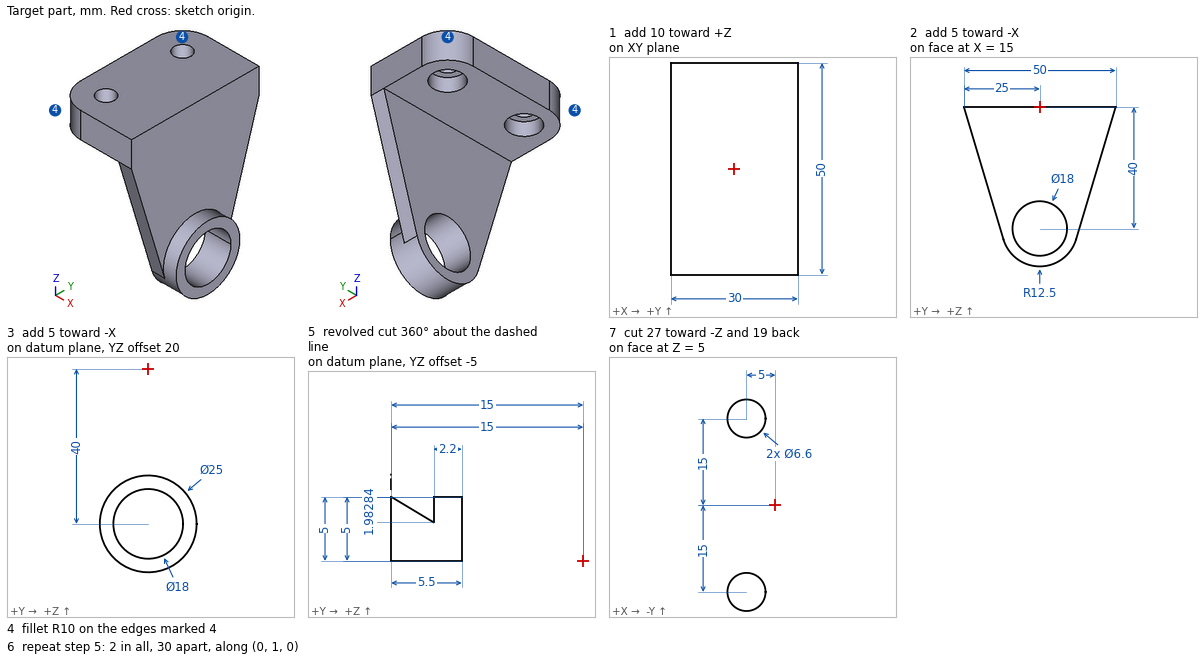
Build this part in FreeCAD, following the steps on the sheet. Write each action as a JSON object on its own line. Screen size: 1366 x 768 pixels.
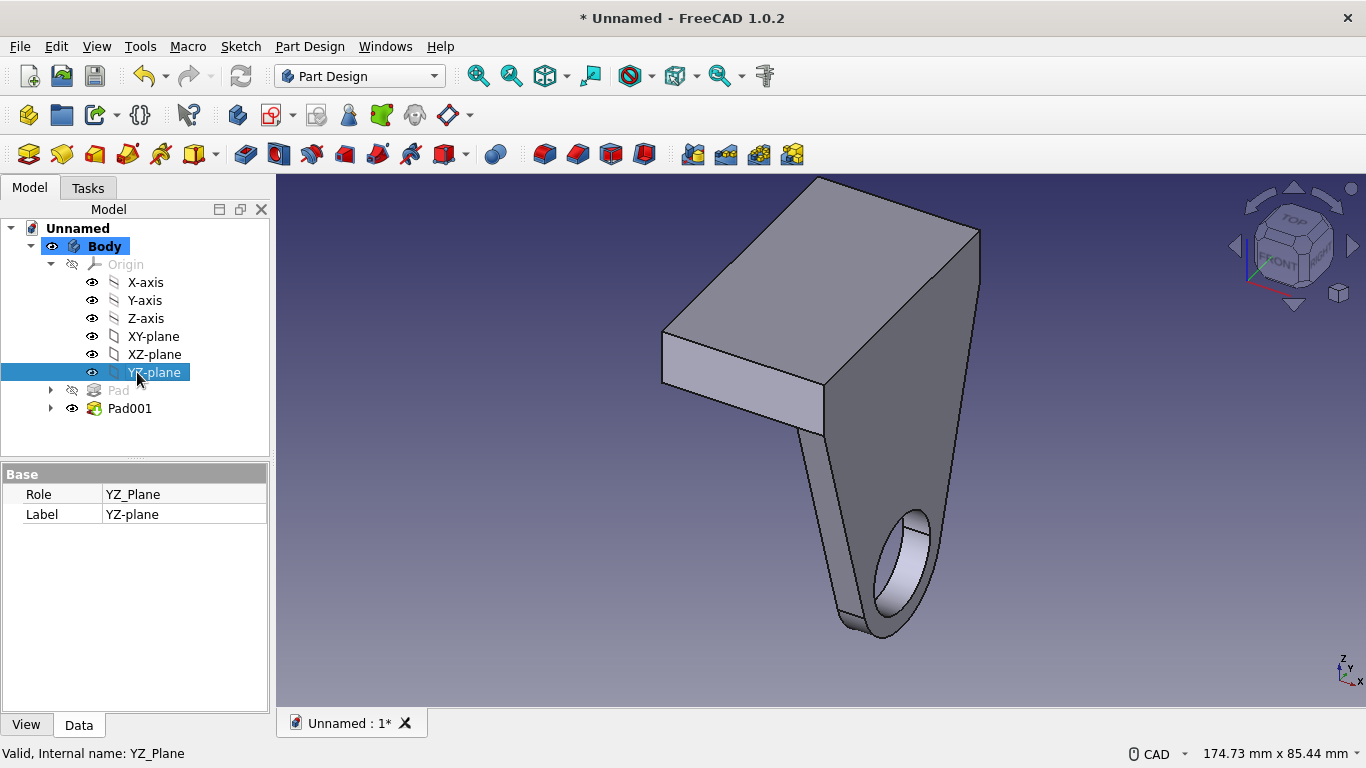
{"action": "left_click", "coordinate": [448, 116]}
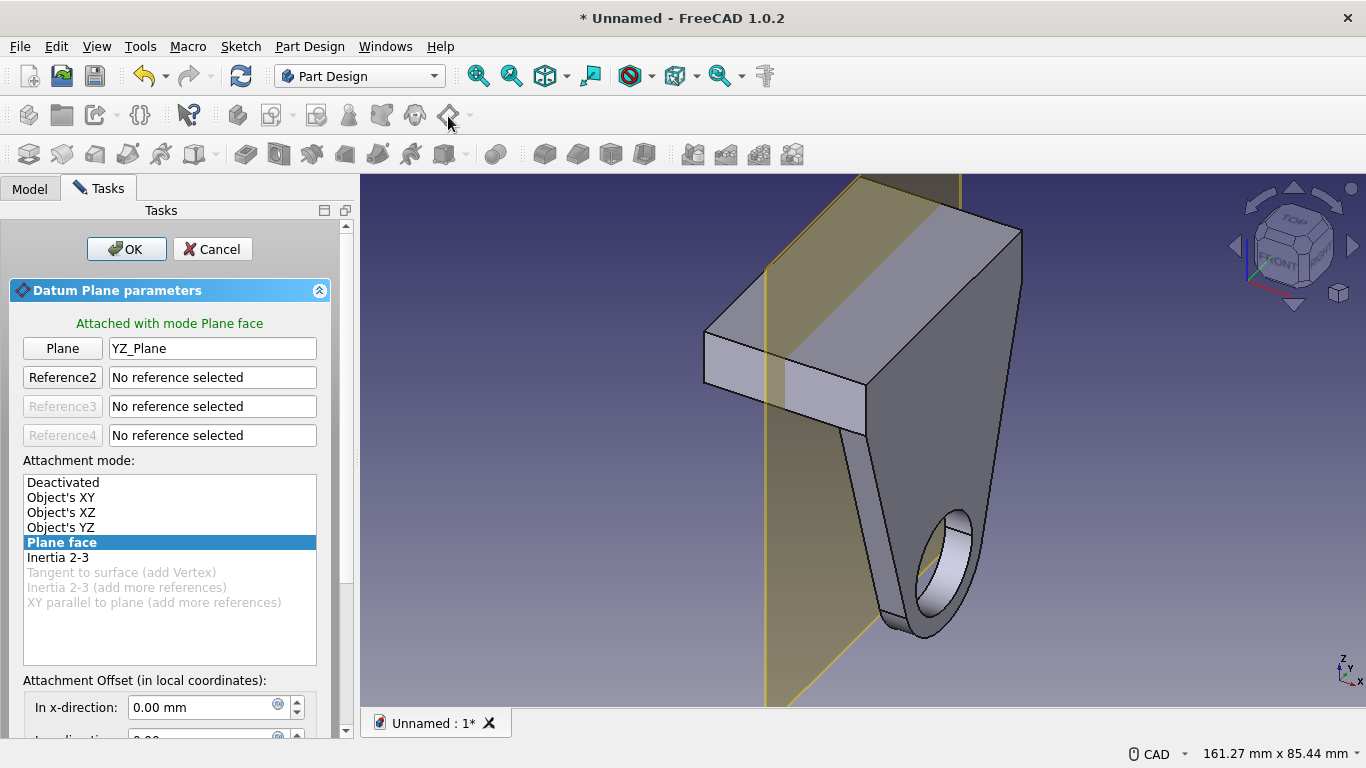
{"action": "scroll", "coordinate": [346, 479], "scroll_direction": "down", "scroll_amount": 2}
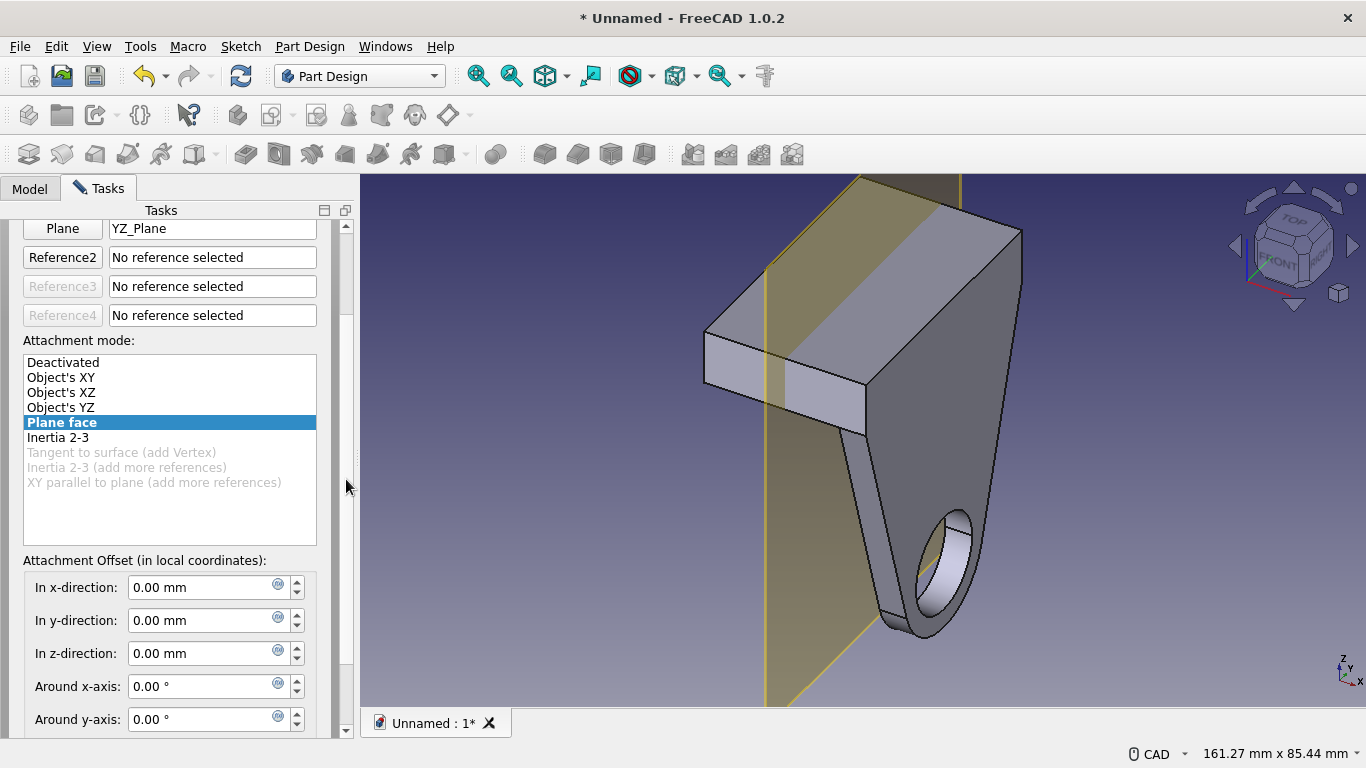
{"action": "triple_click", "coordinate": [210, 654]}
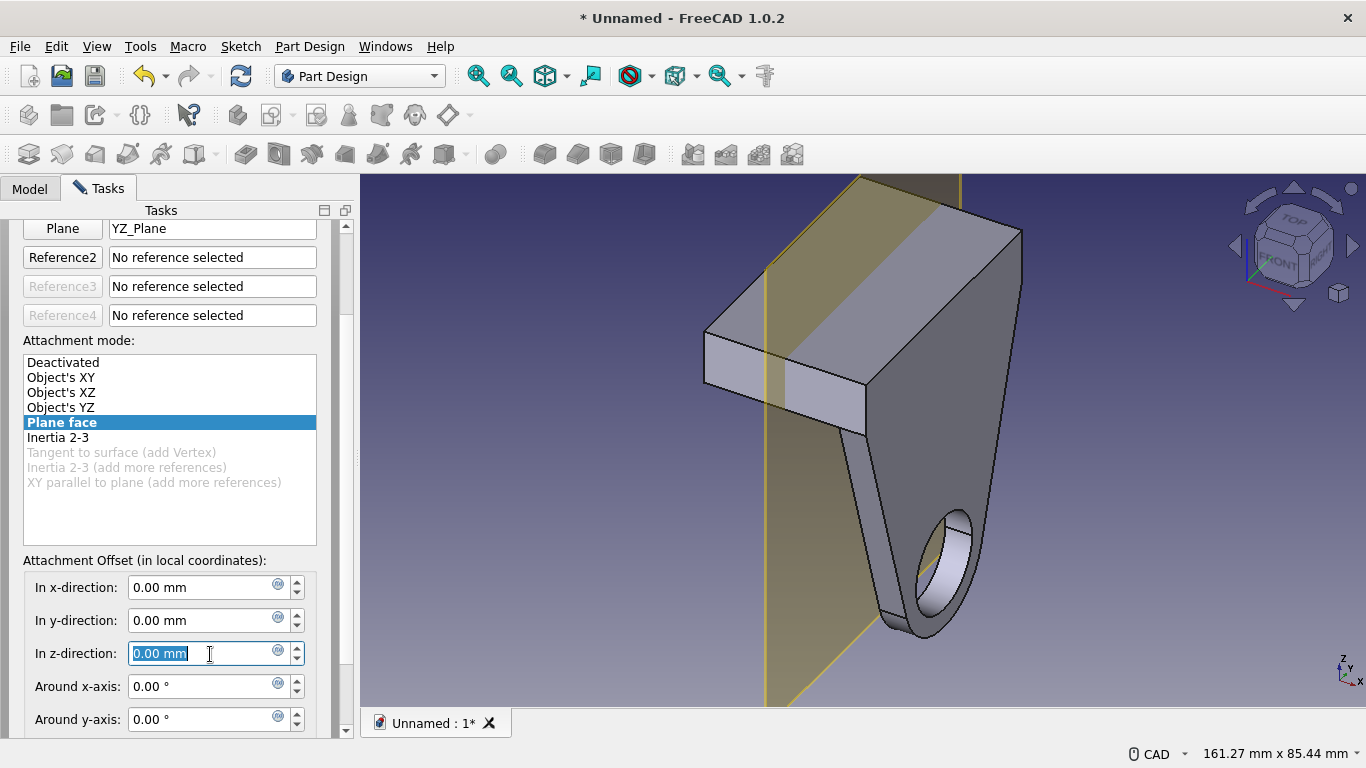
{"action": "type", "text": "20"}
{"action": "key", "text": "Tab"}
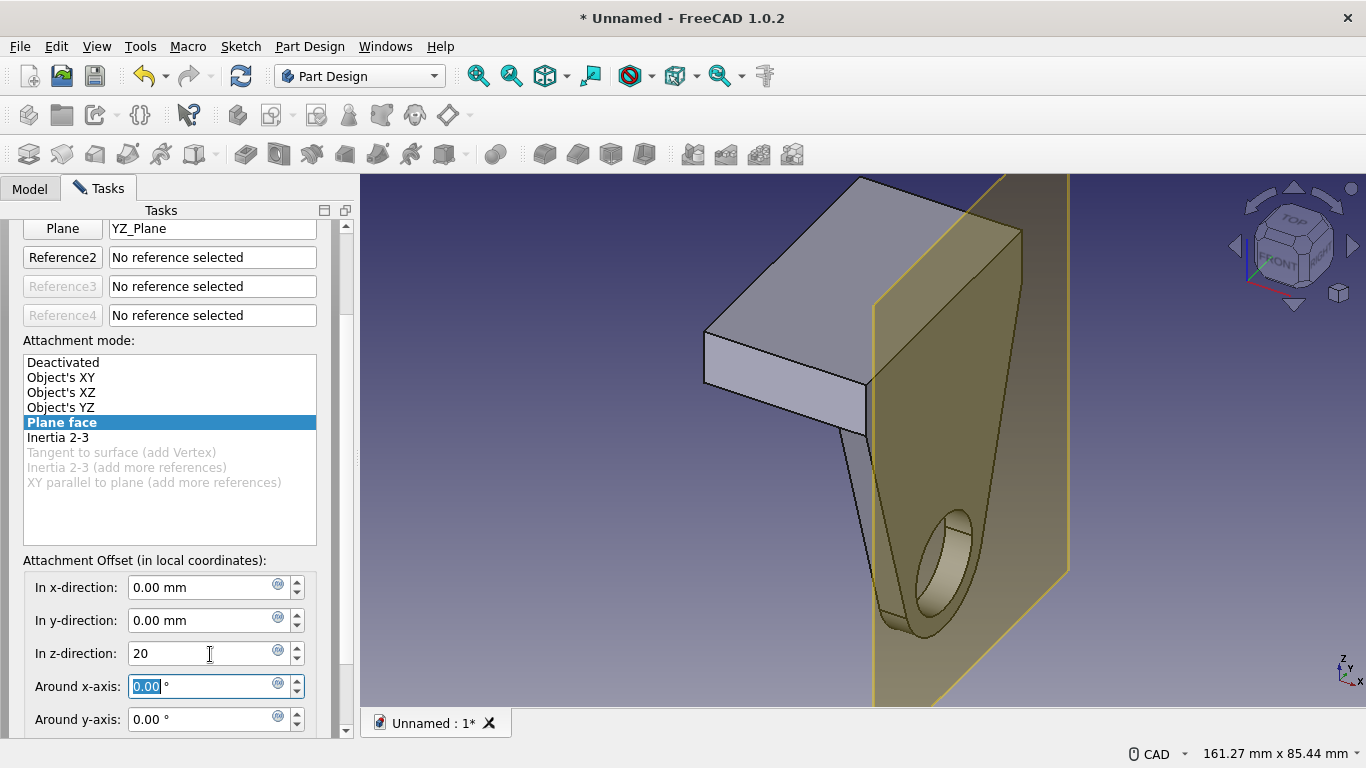
{"action": "scroll", "coordinate": [346, 479], "scroll_direction": "up", "scroll_amount": 3}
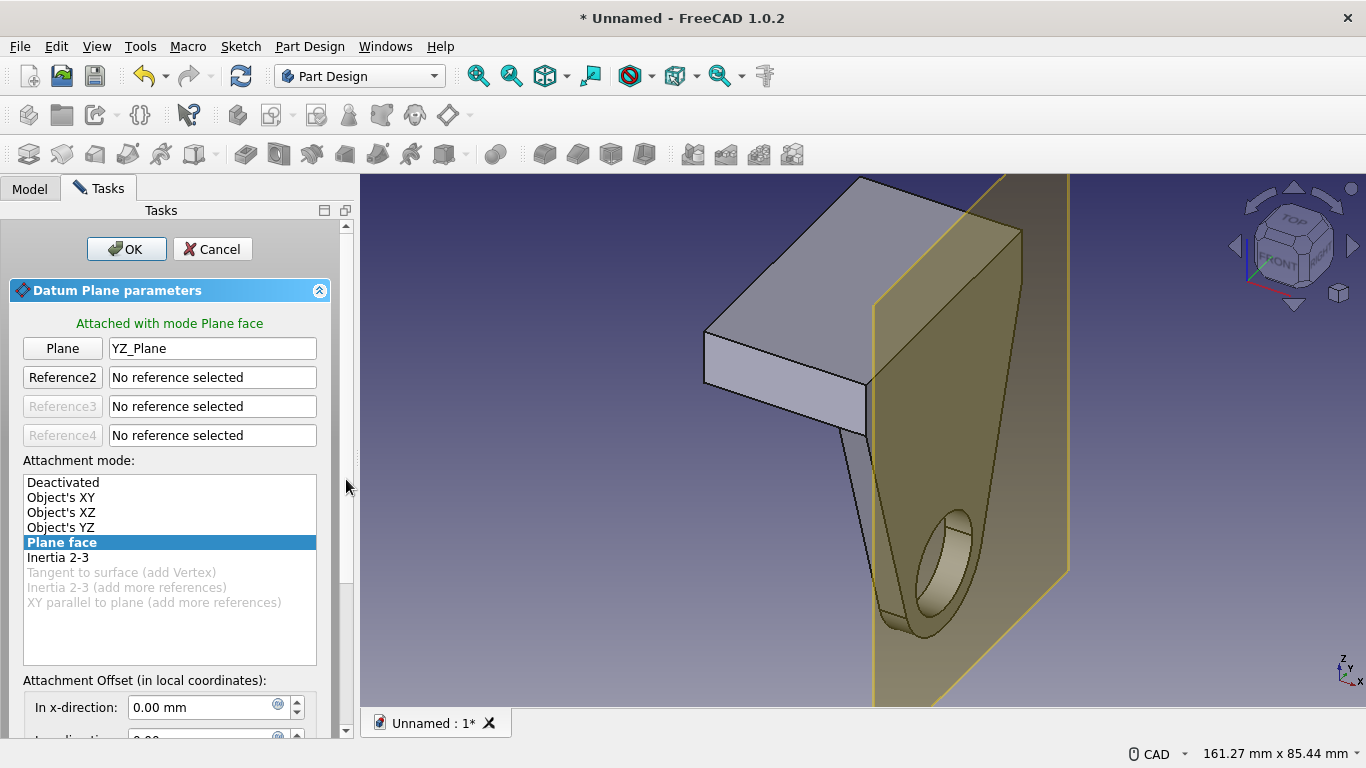
{"action": "left_click", "coordinate": [127, 249]}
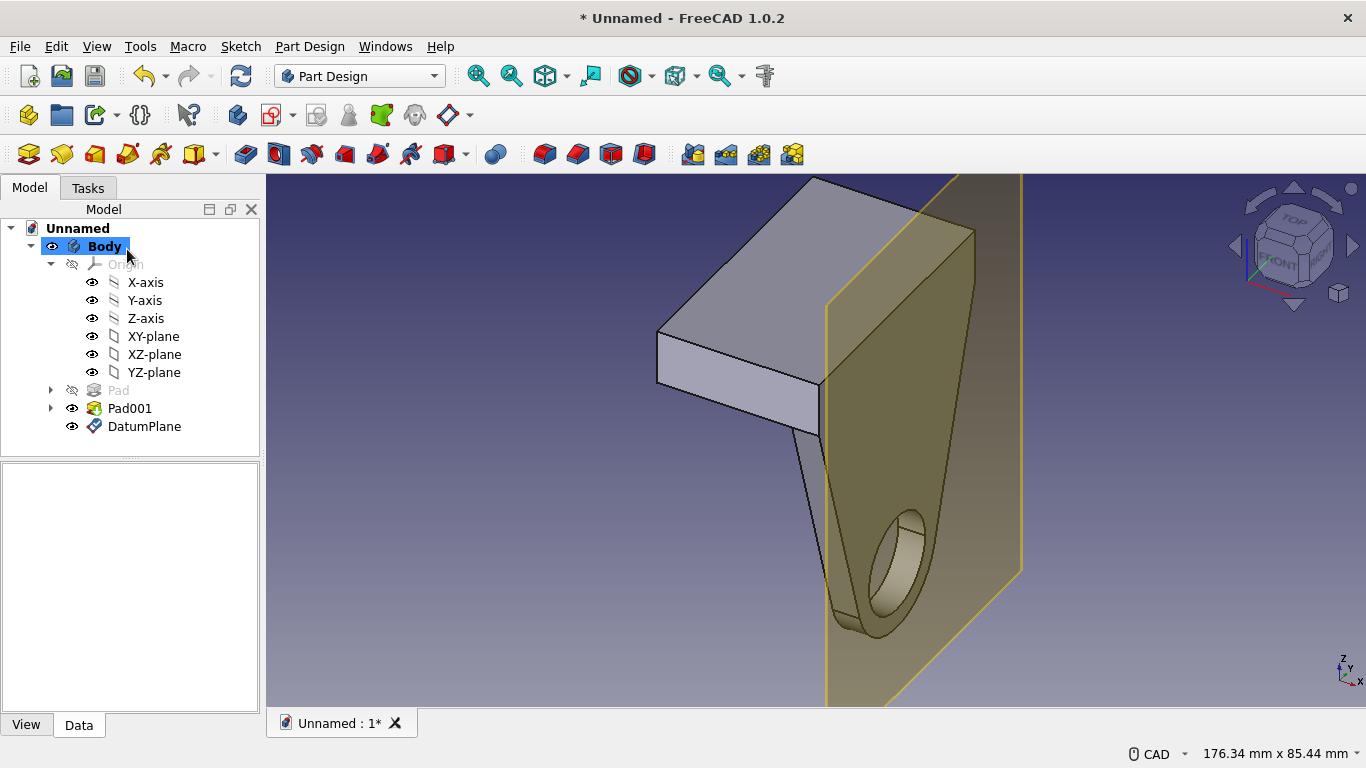
{"action": "left_click", "coordinate": [117, 426]}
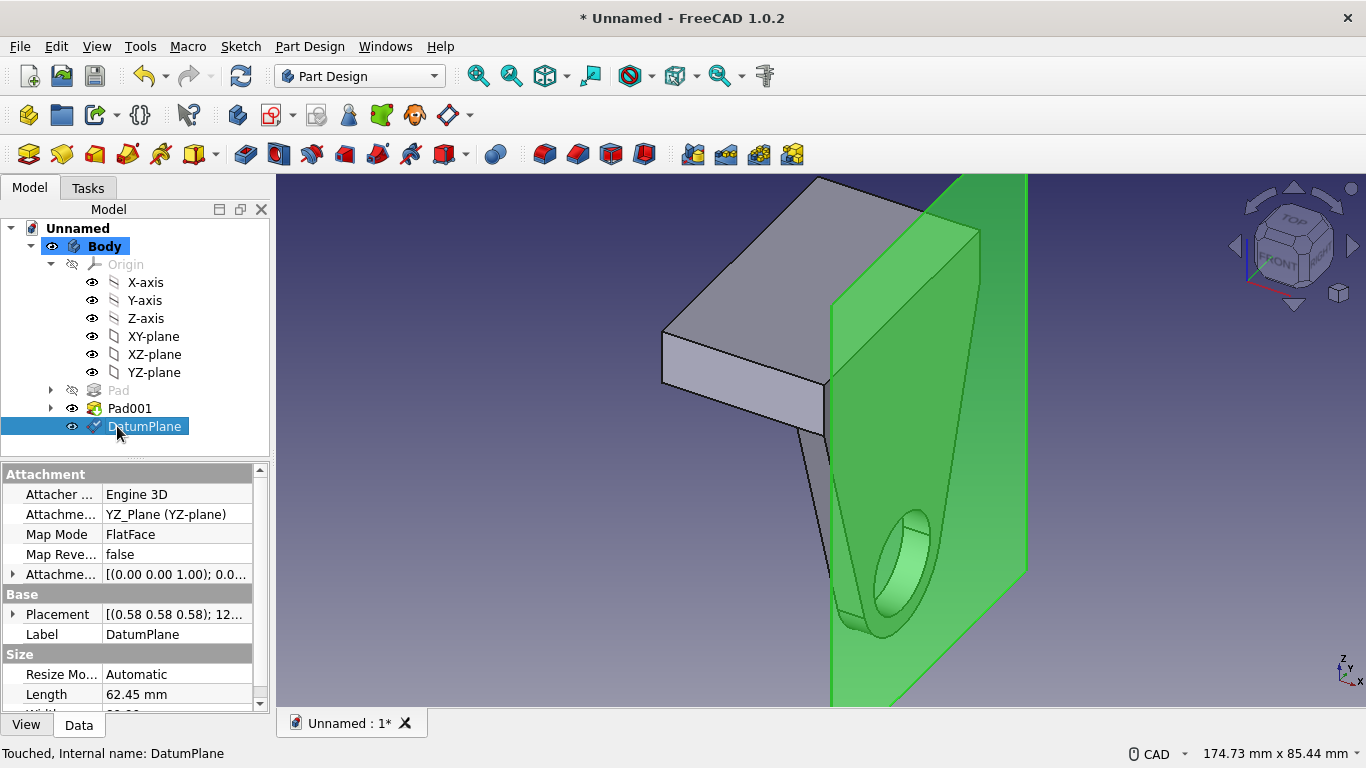
{"action": "left_click", "coordinate": [270, 116]}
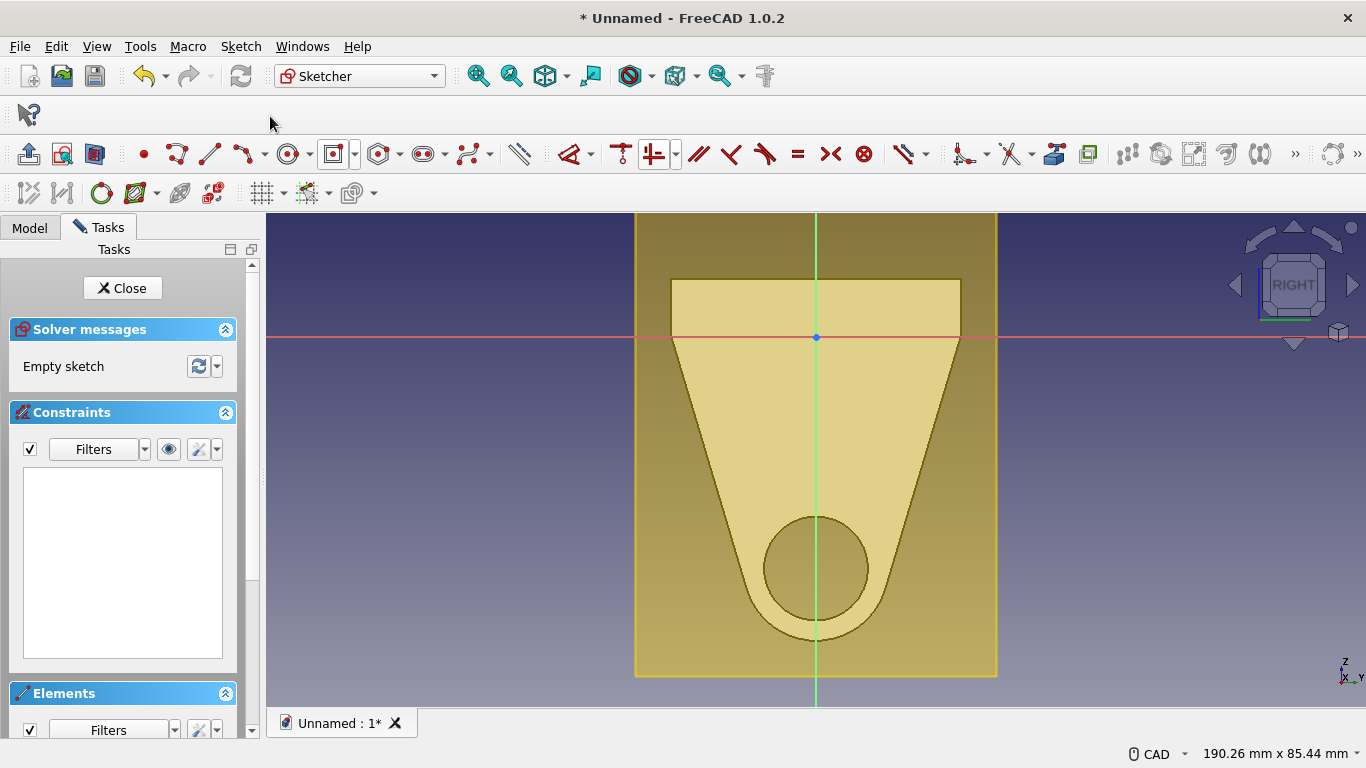
{"action": "left_click", "coordinate": [288, 154]}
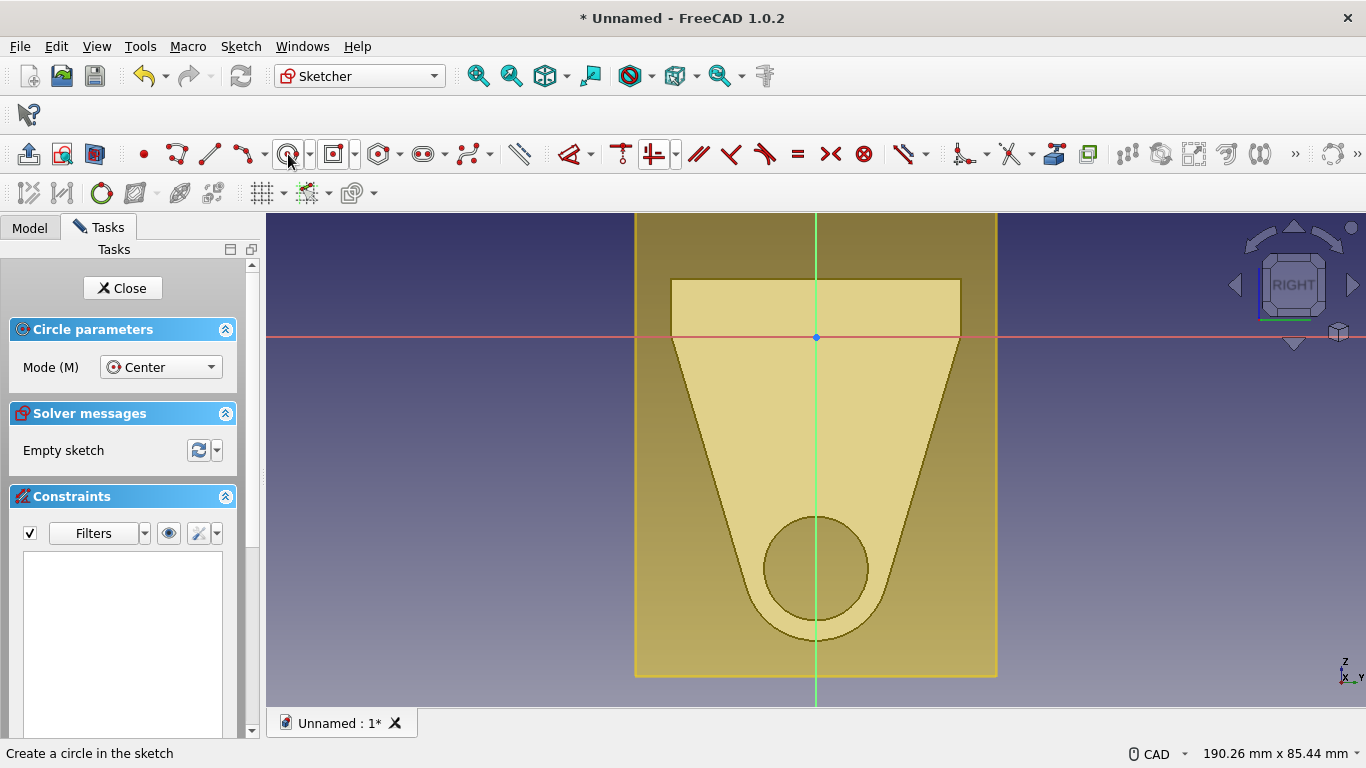
{"action": "left_click", "coordinate": [816, 569]}
{"action": "mouse_move", "coordinate": [867, 517]}